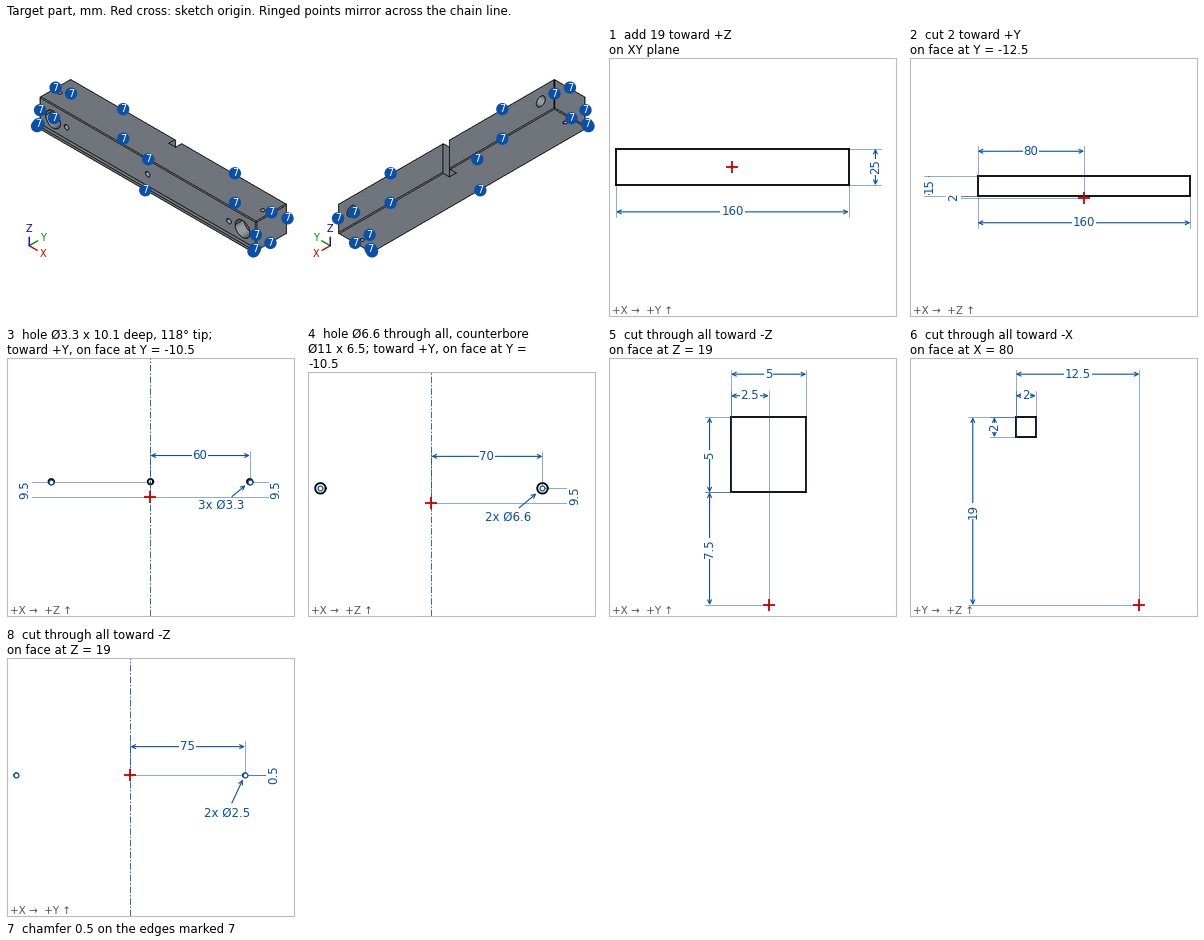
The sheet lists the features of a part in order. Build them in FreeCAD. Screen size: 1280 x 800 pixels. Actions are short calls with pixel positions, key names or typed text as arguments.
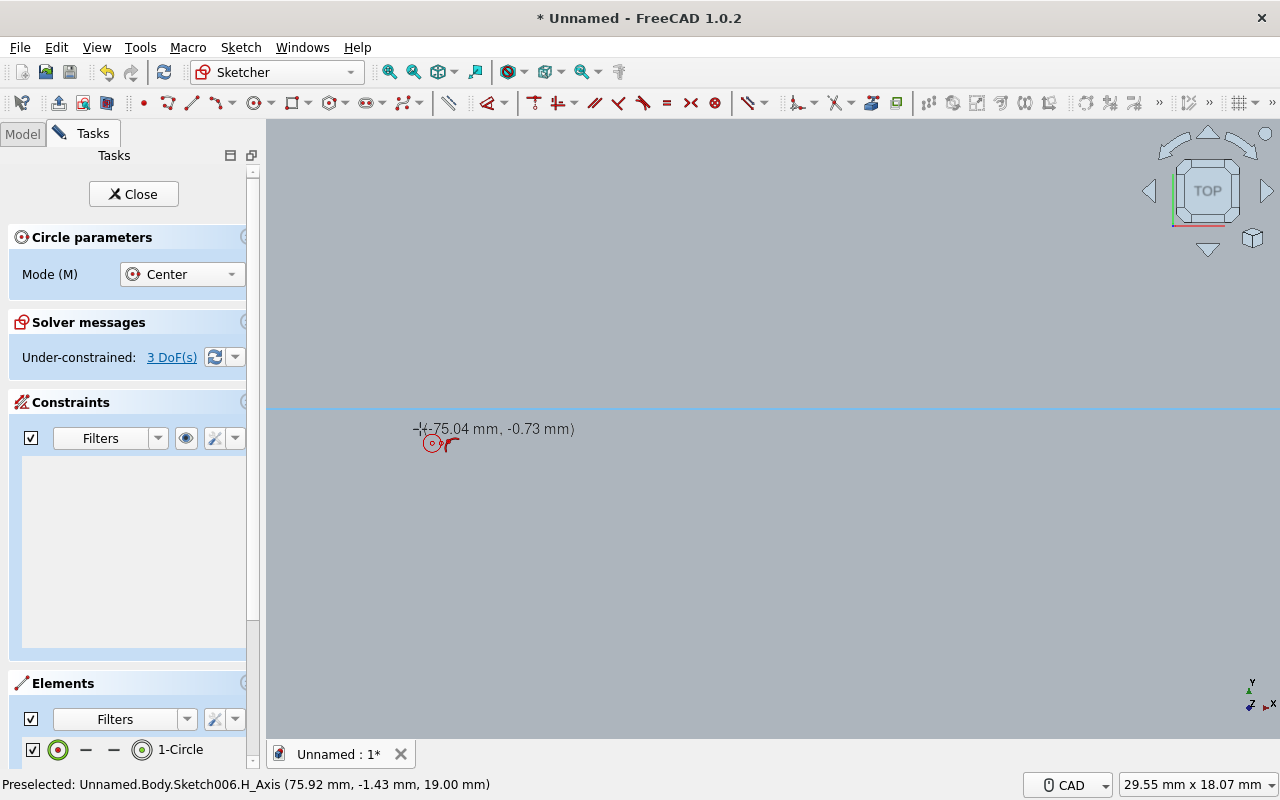
click(420, 426)
click(451, 456)
key(Escape)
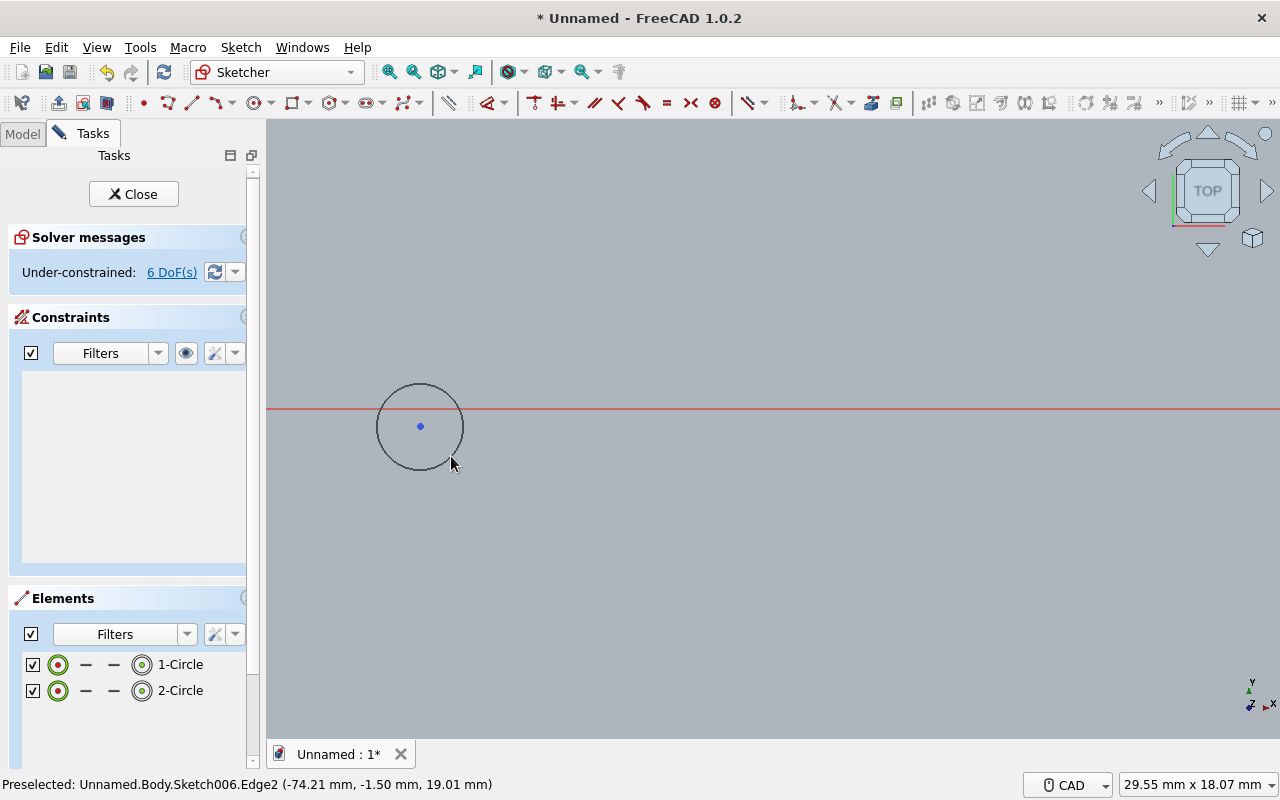
scroll(419, 429, down, 11)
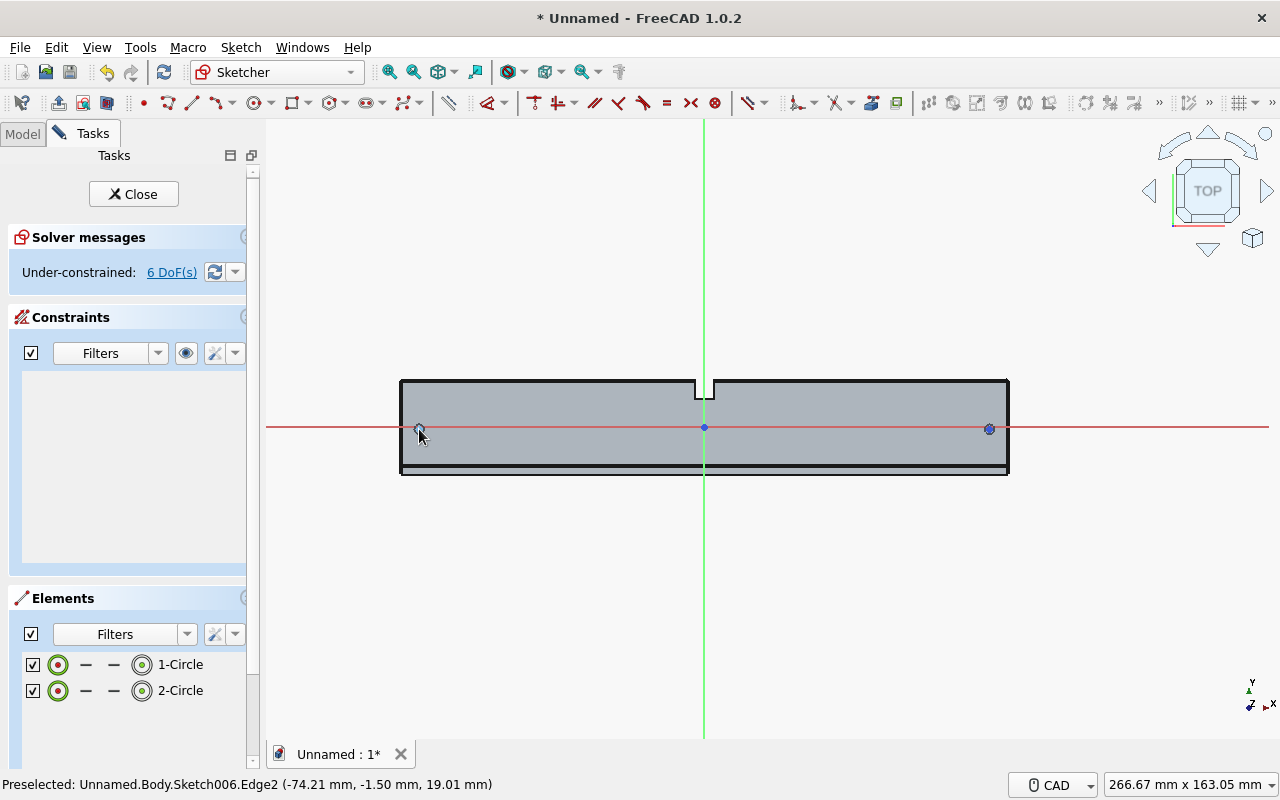
scroll(993, 426, up, 12)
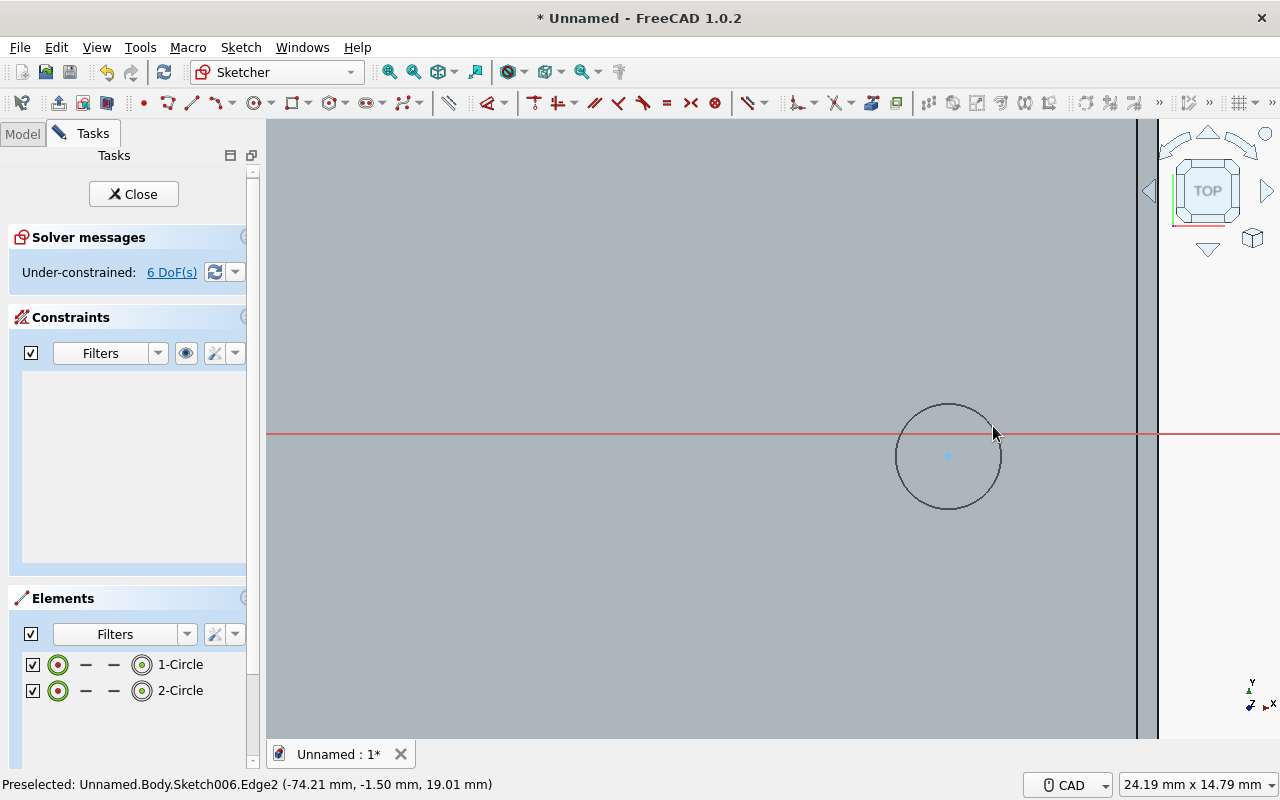
click(986, 419)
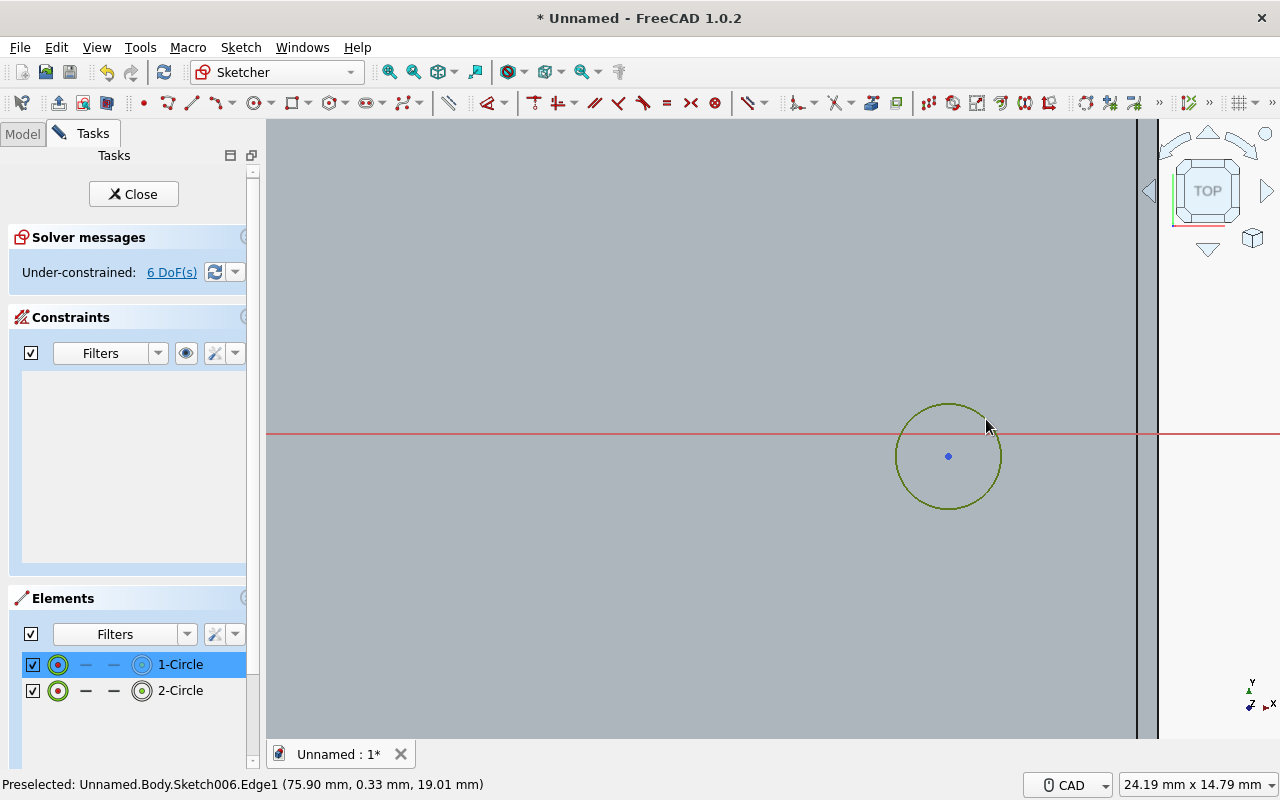
scroll(994, 426, down, 12)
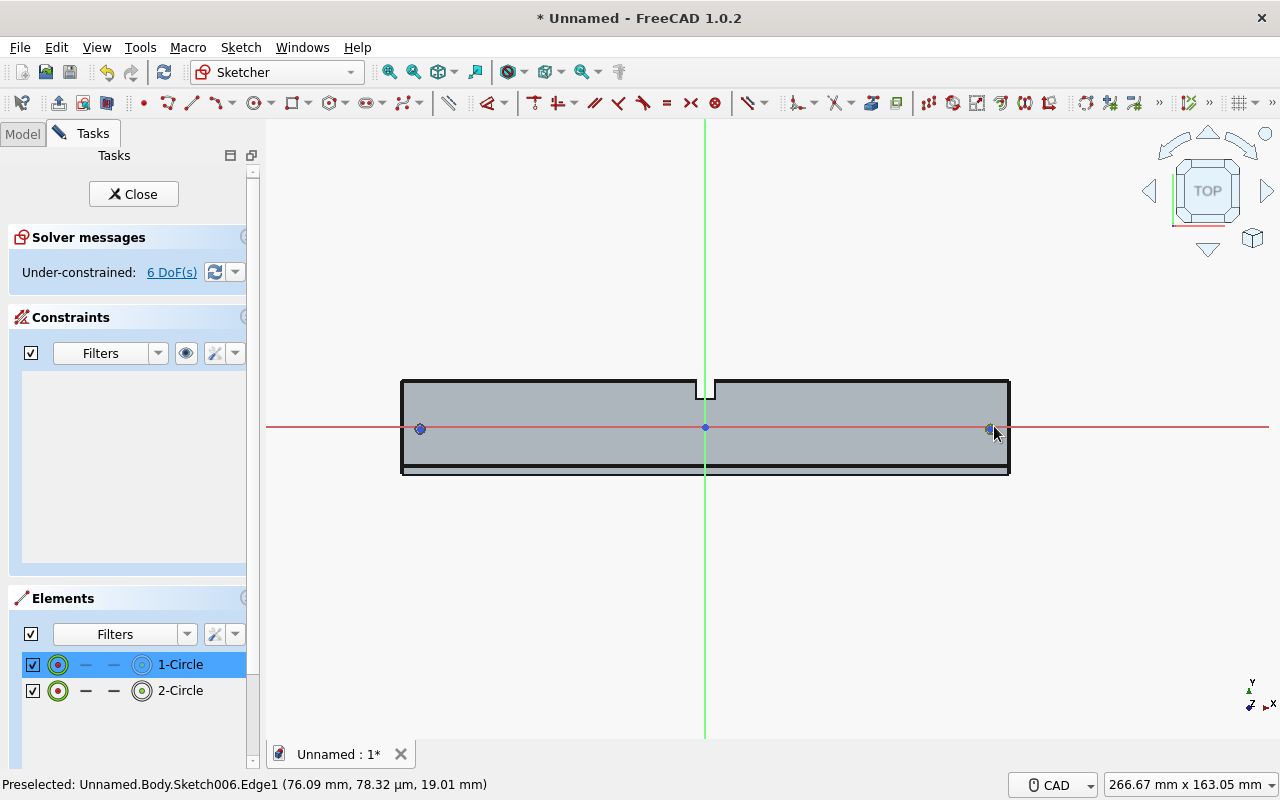
scroll(424, 426, up, 12)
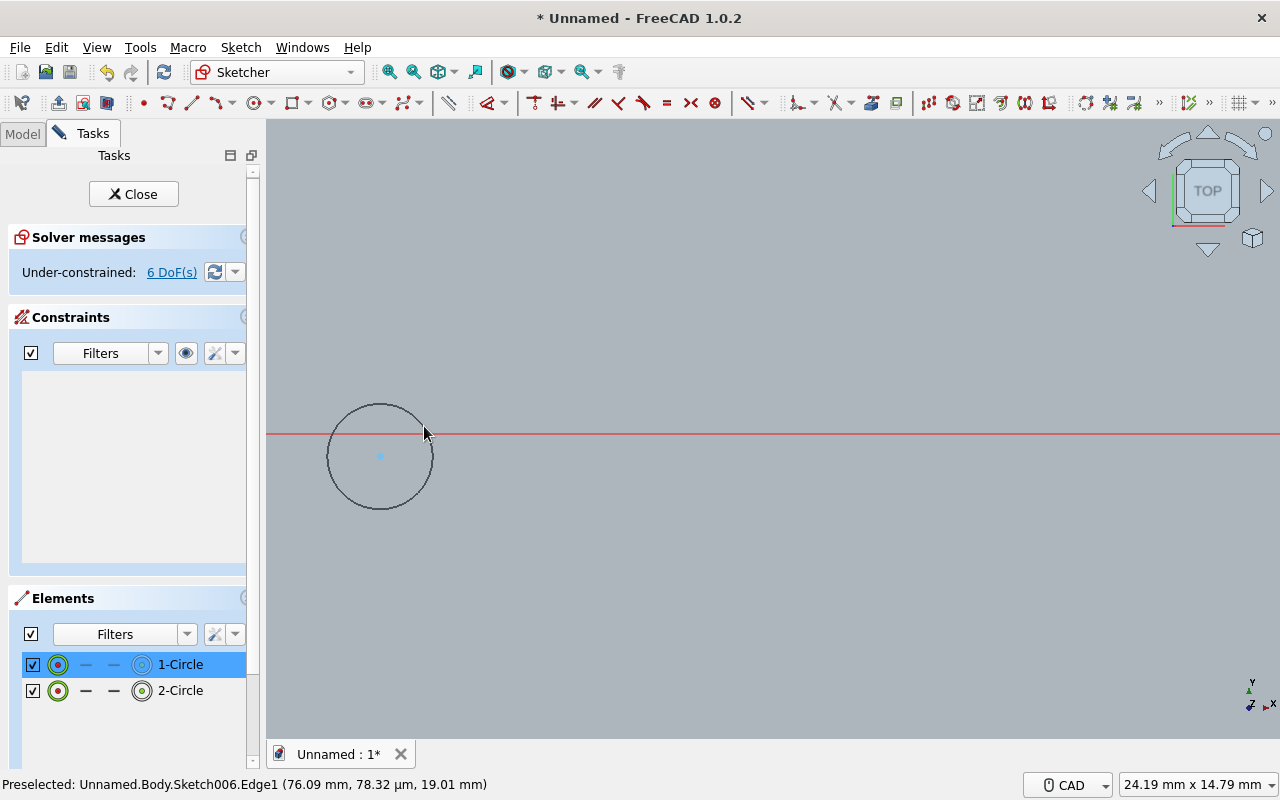
click(417, 419)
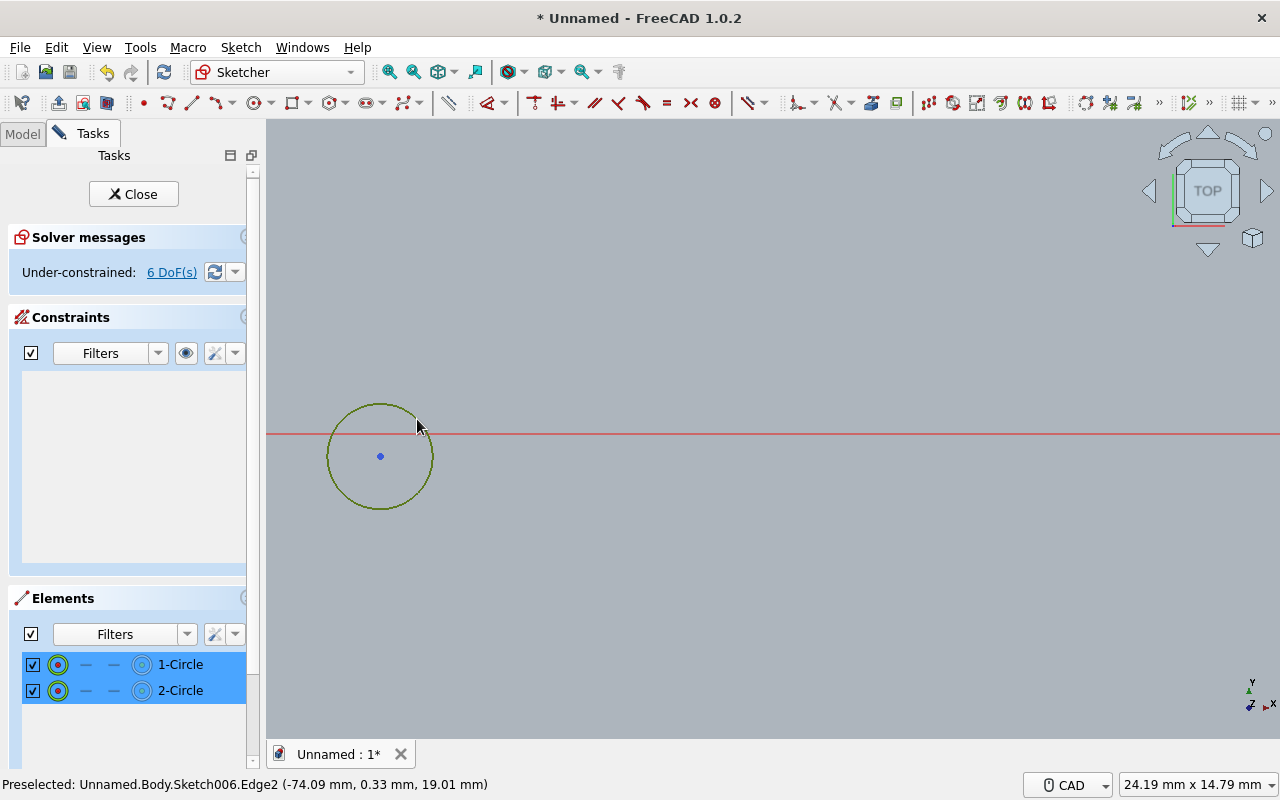
key(e)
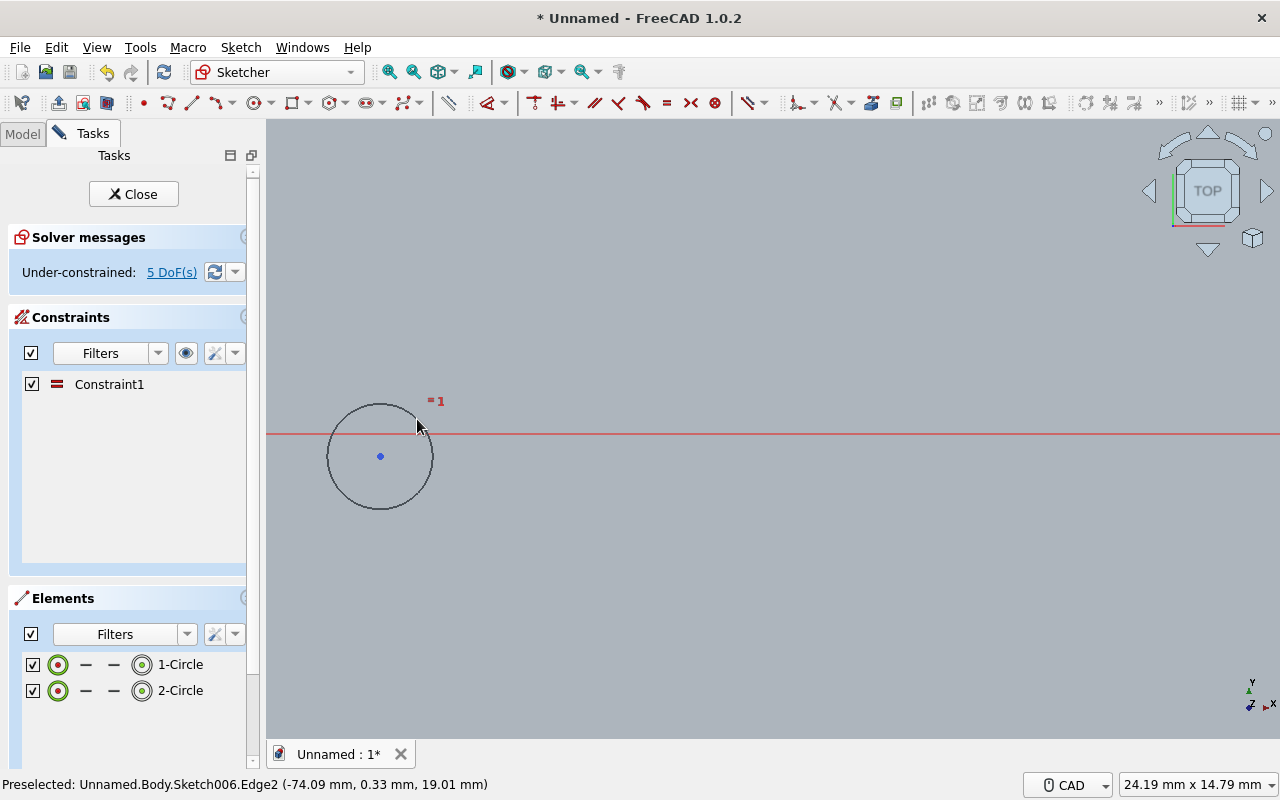
scroll(423, 426, down, 12)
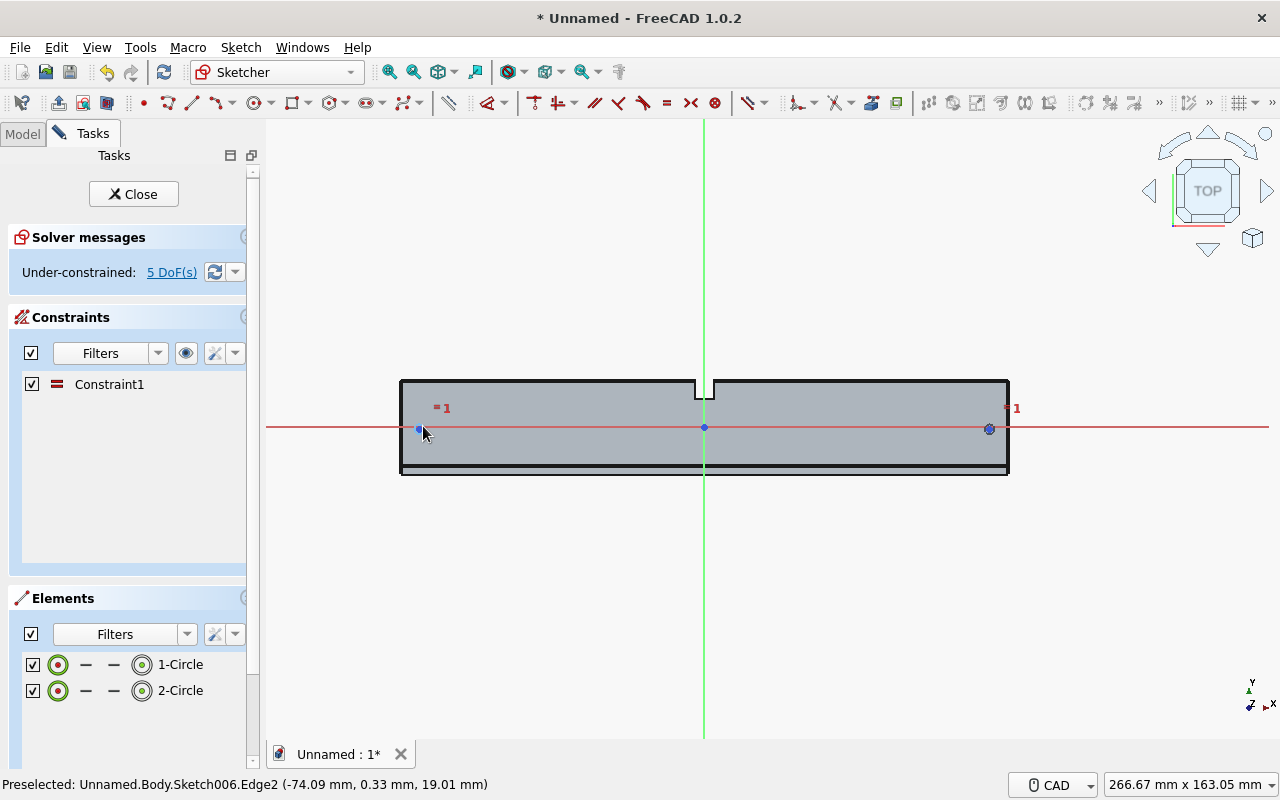
click(990, 429)